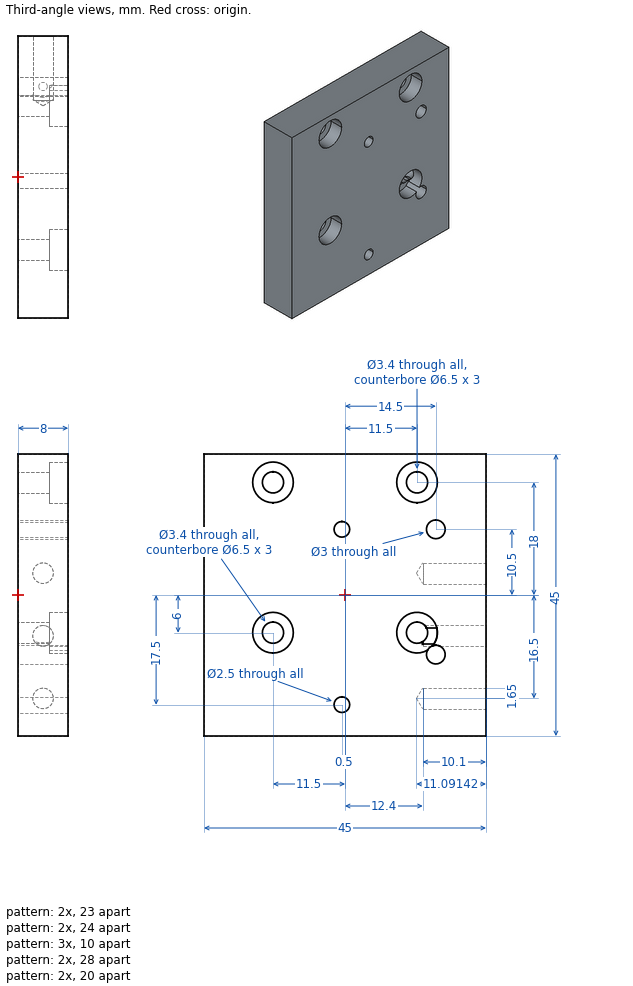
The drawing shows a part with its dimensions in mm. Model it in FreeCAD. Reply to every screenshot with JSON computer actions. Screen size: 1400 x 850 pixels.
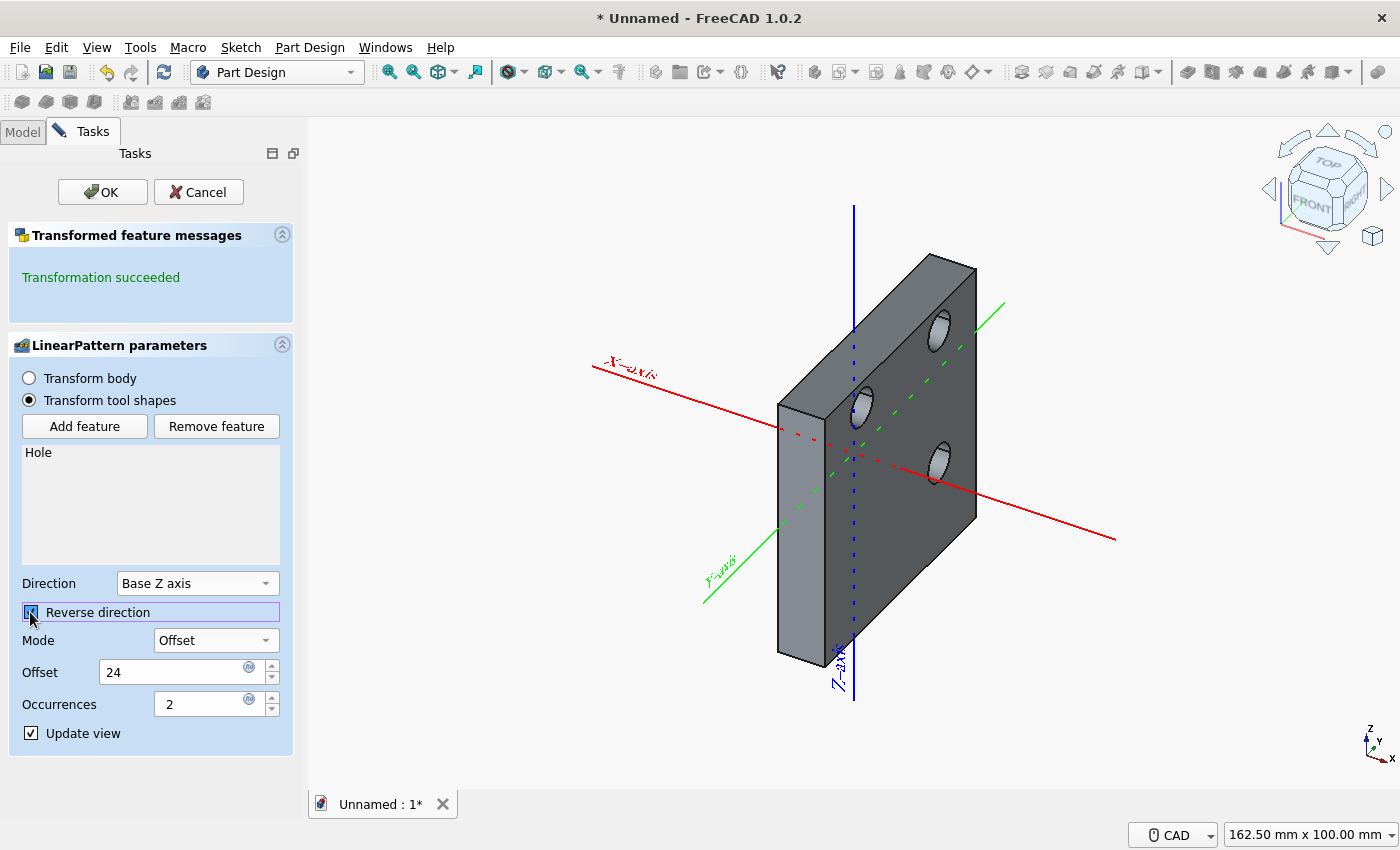
{"action": "left_click", "coordinate": [103, 192]}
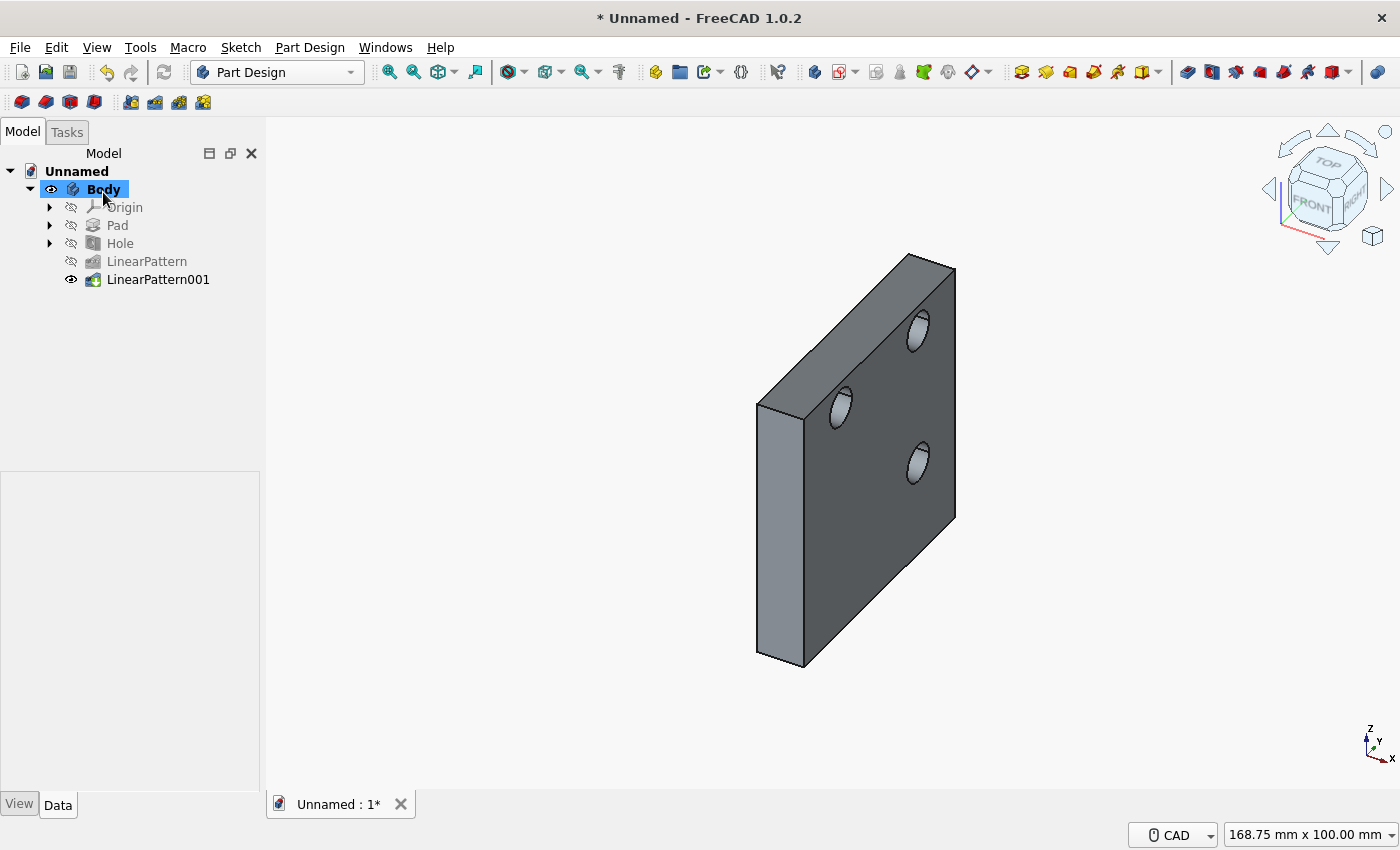
{"action": "left_click", "coordinate": [858, 489]}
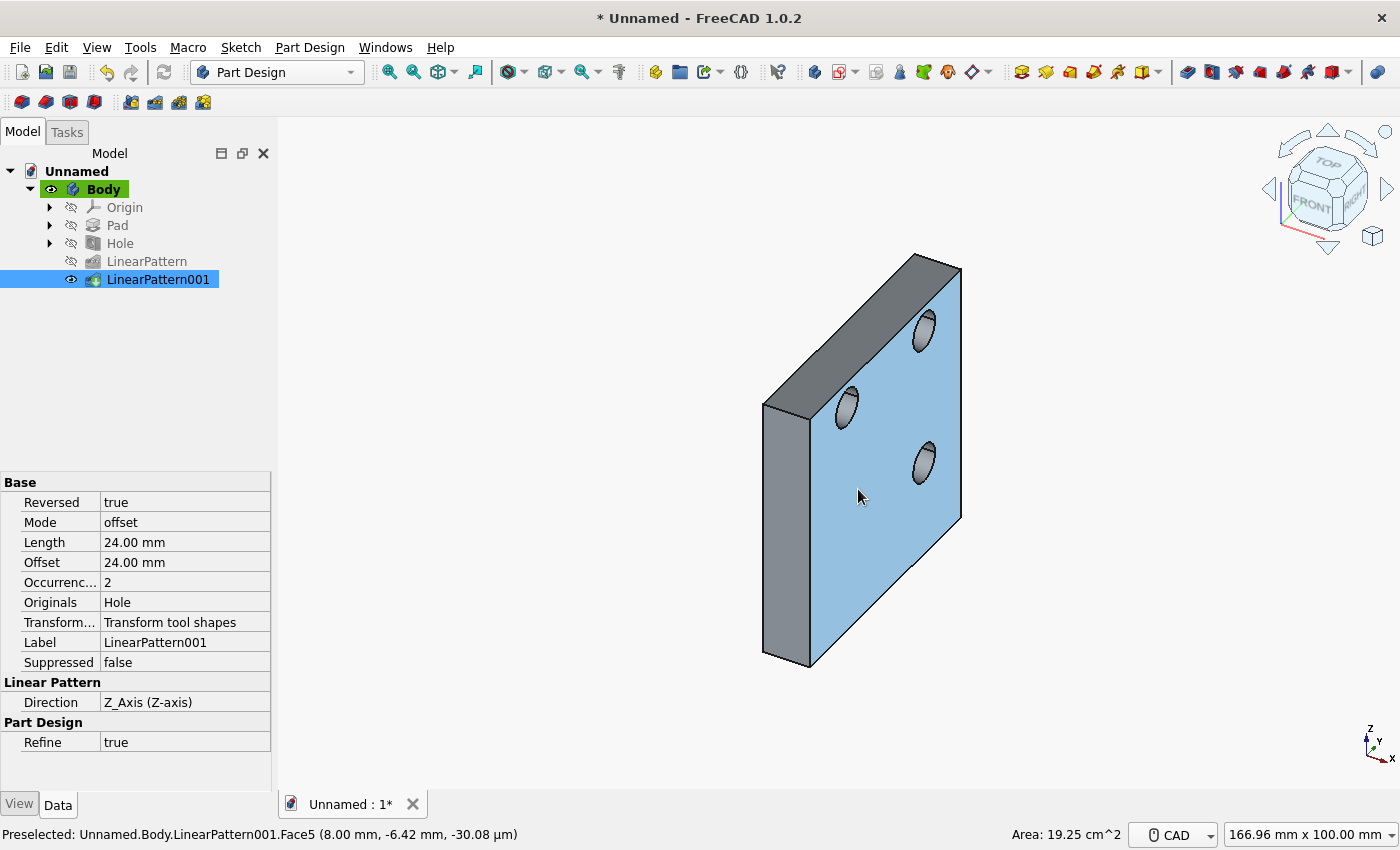
{"action": "left_click", "coordinate": [840, 72]}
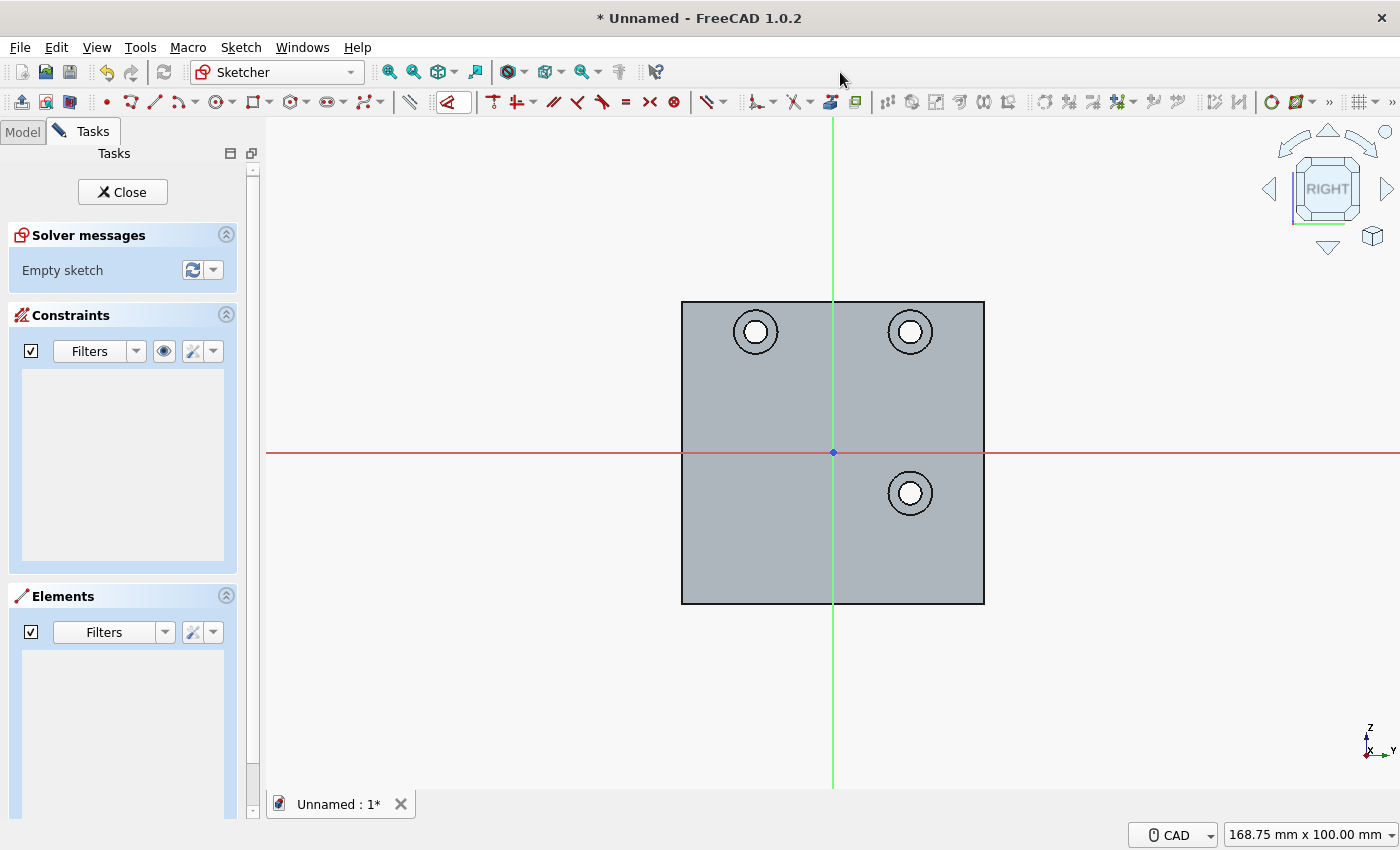
{"action": "scroll", "coordinate": [755, 495], "scroll_direction": "up", "scroll_amount": 15}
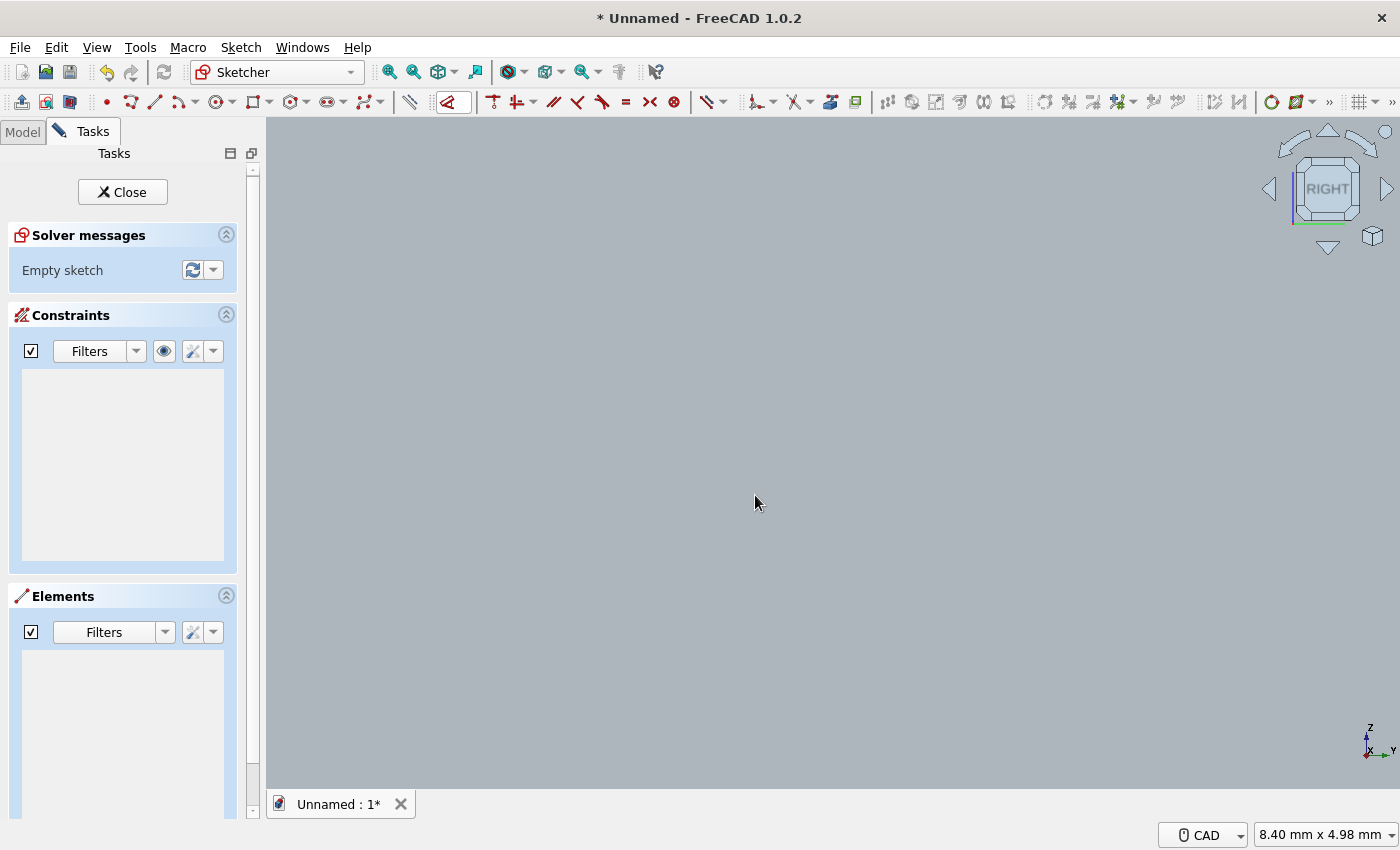
{"action": "key", "text": "g c"}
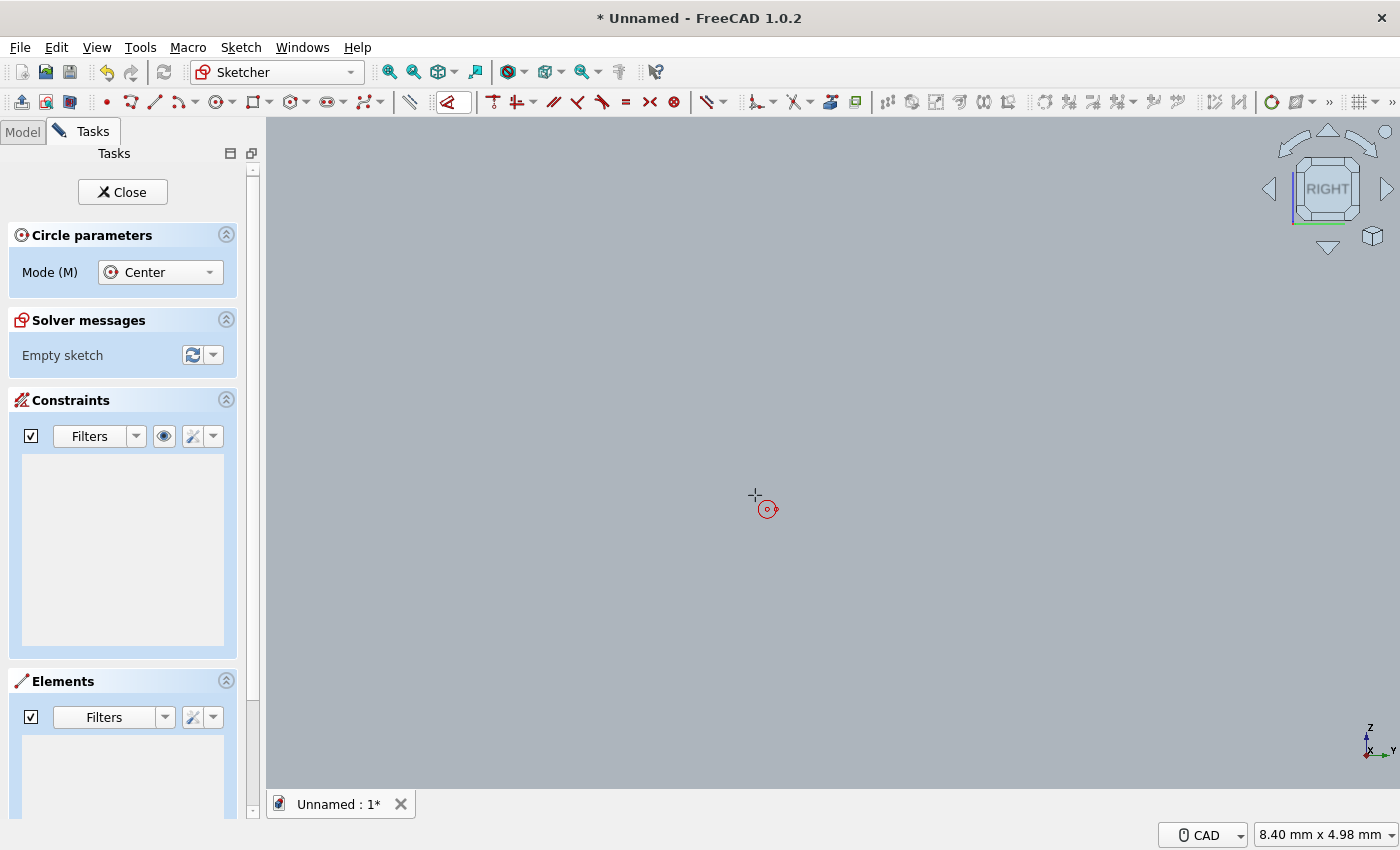
{"action": "left_click", "coordinate": [761, 451]}
{"action": "left_click", "coordinate": [923, 288]}
{"action": "key", "text": "Escape"}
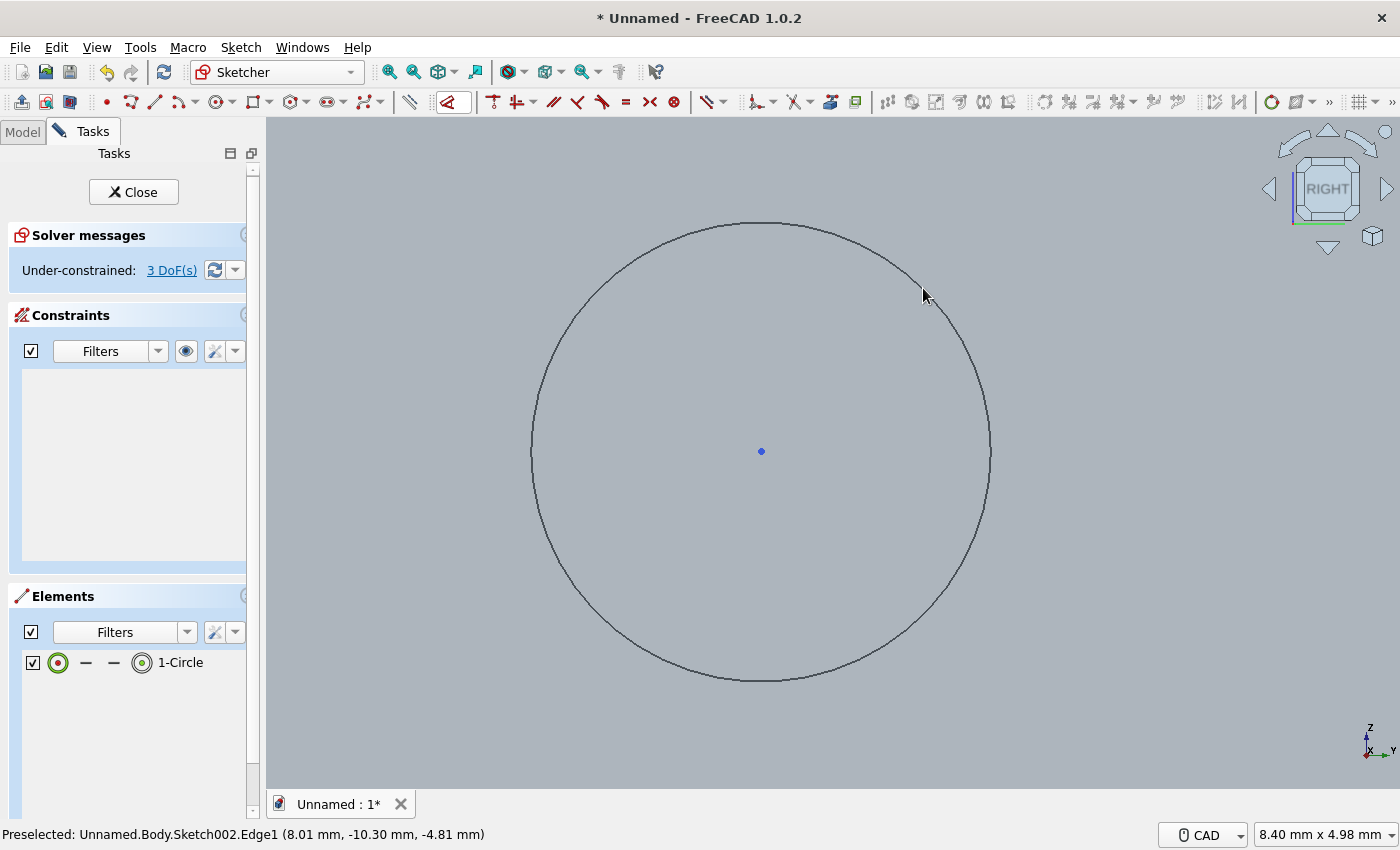
{"action": "key", "text": "d"}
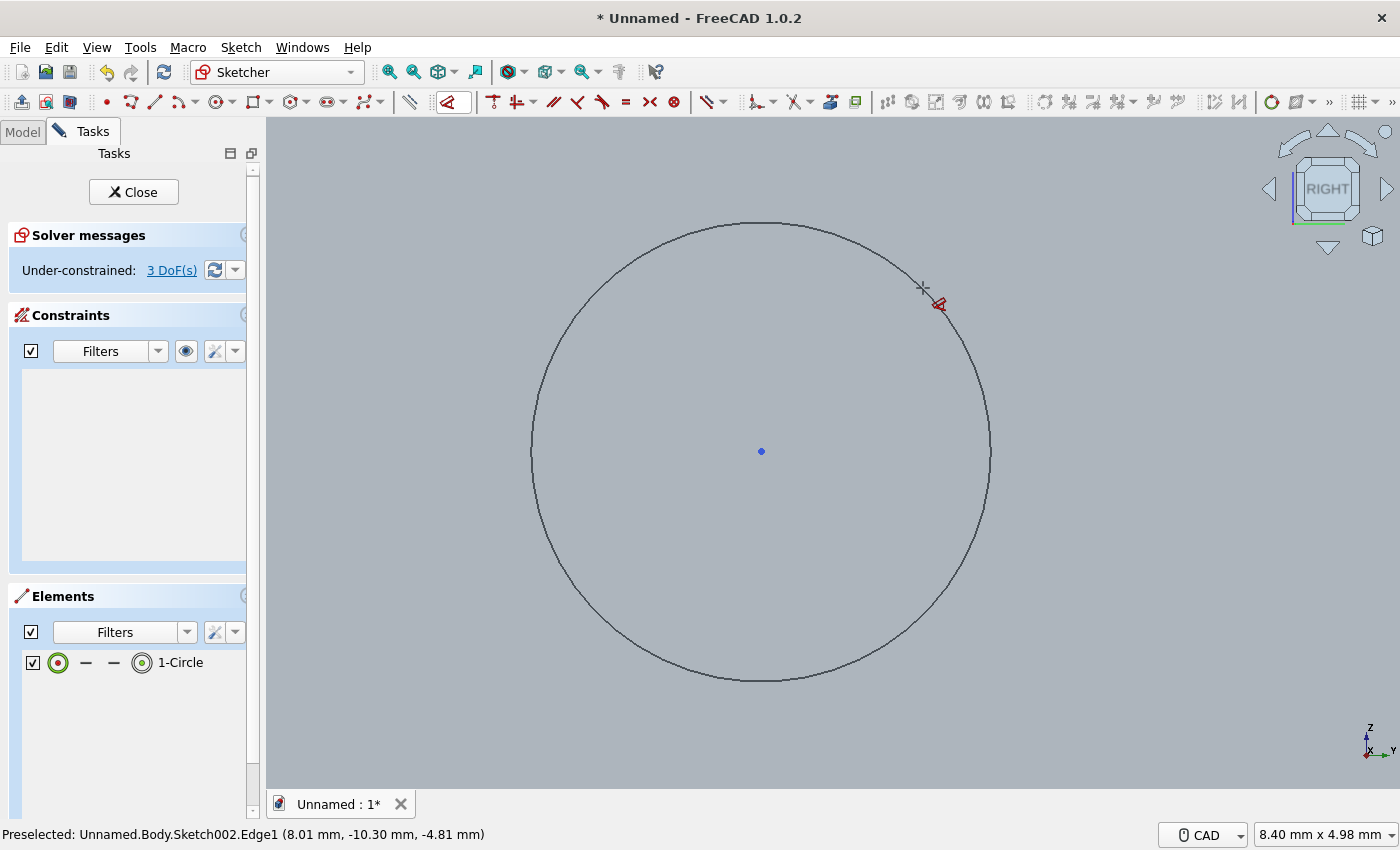
{"action": "left_click", "coordinate": [923, 289]}
{"action": "left_click", "coordinate": [946, 266]}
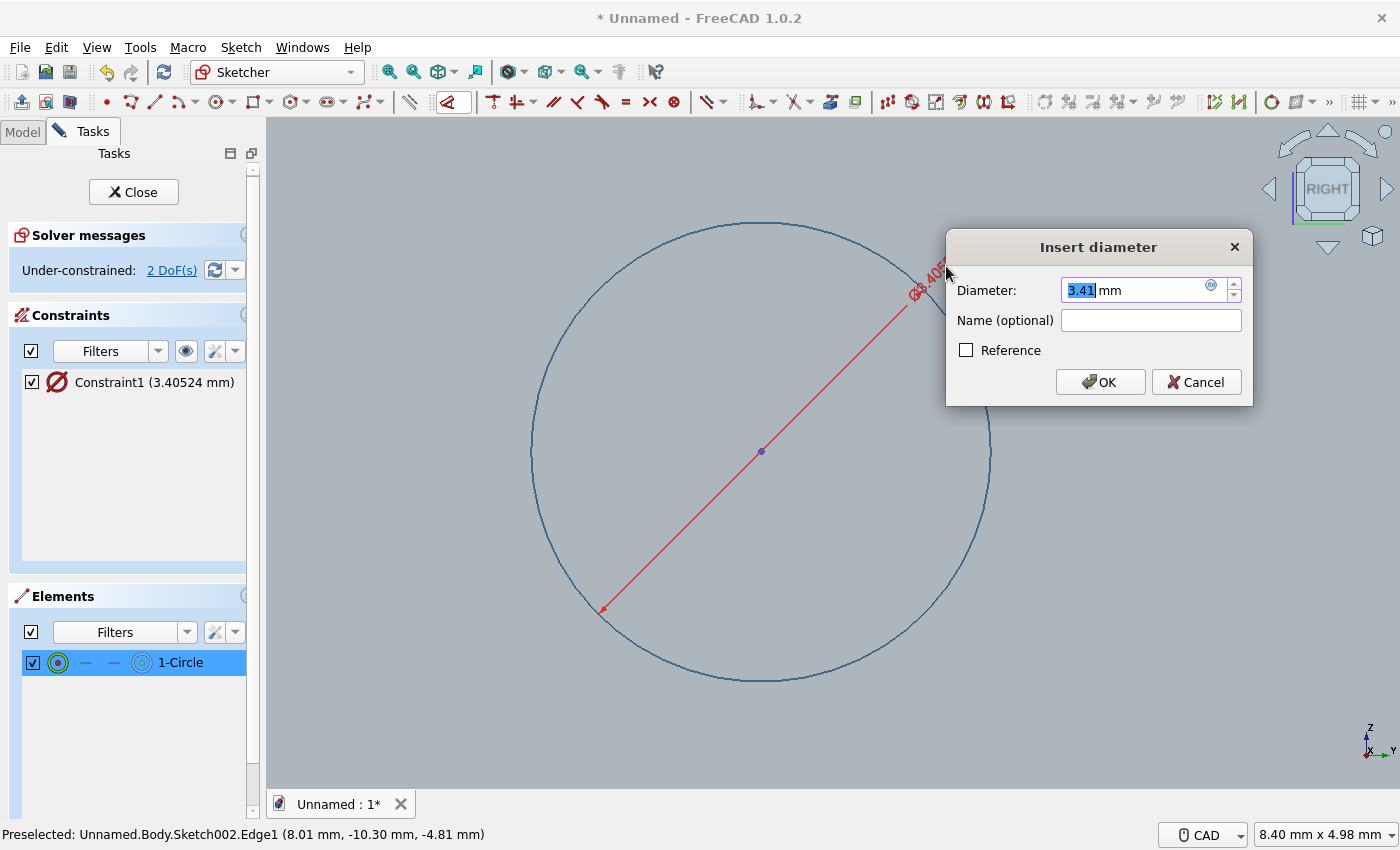
{"action": "type", "text": "3.4"}
{"action": "key", "text": "Return"}